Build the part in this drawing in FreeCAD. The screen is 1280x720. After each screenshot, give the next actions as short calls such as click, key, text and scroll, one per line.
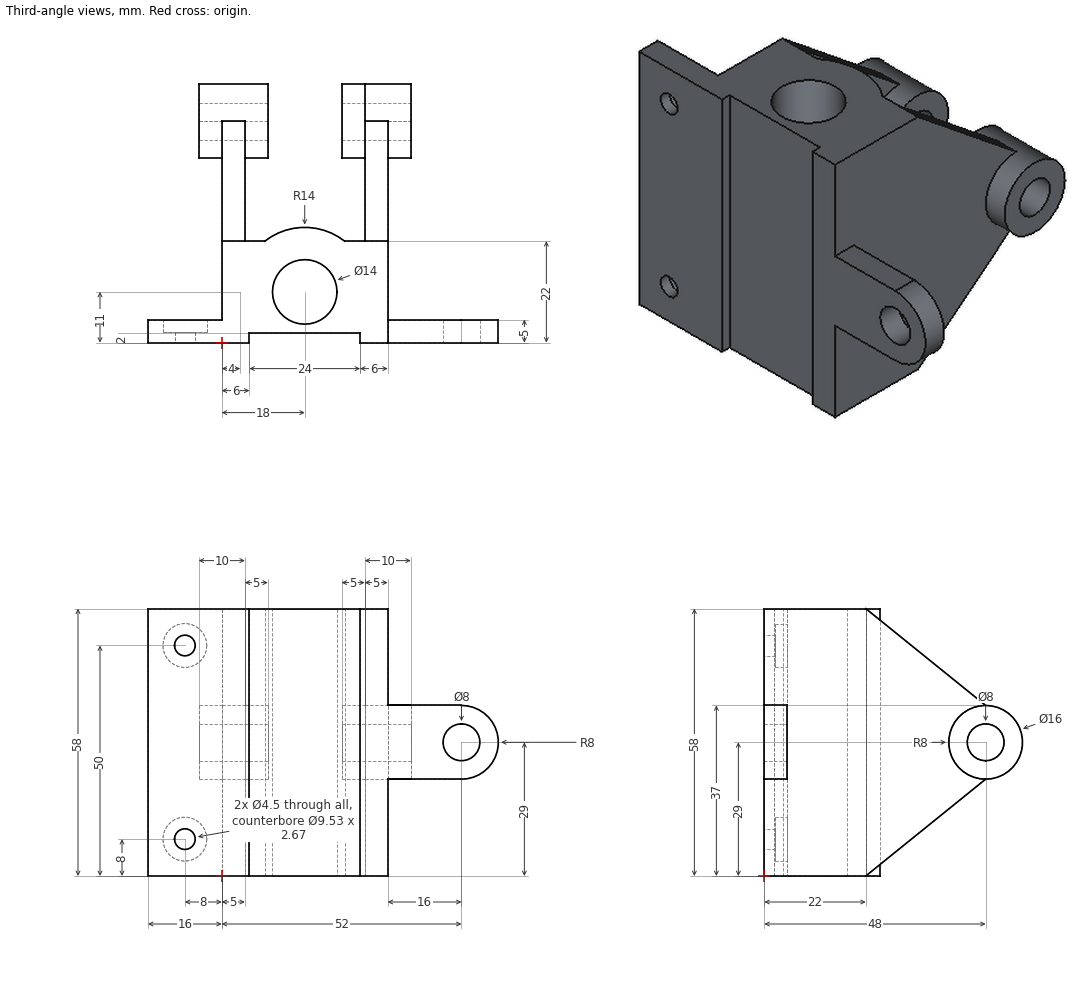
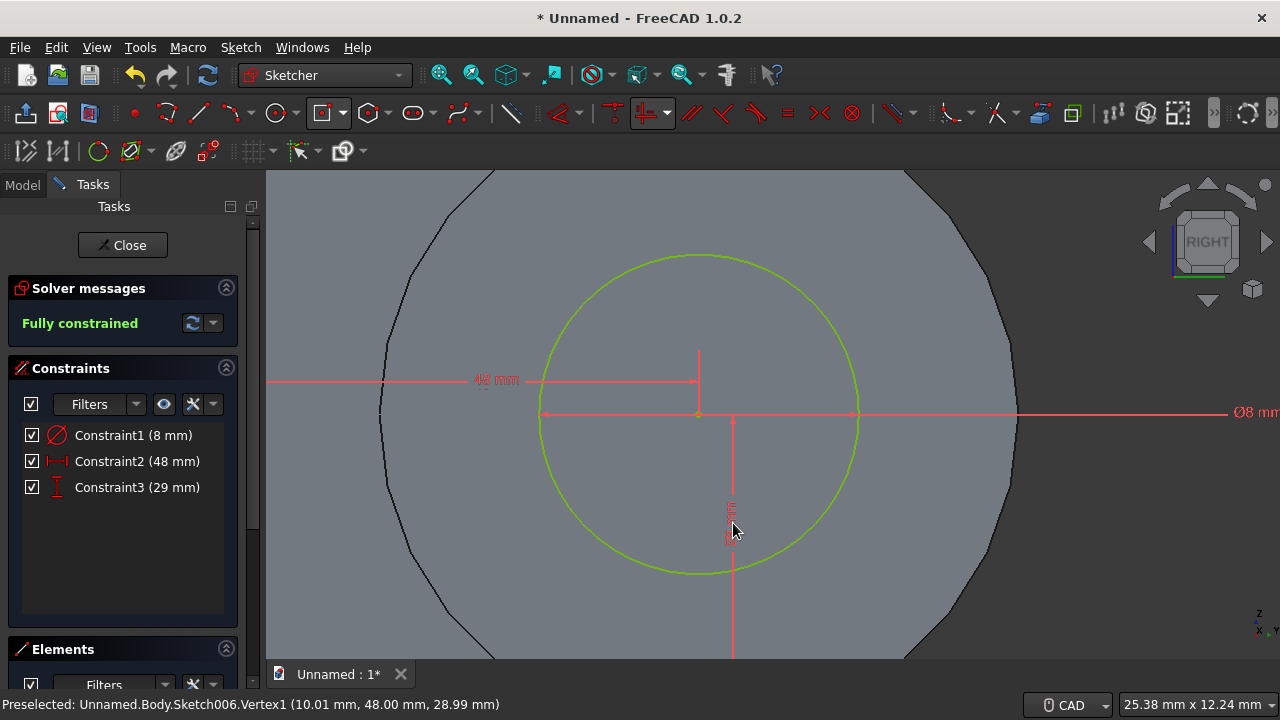
click(123, 245)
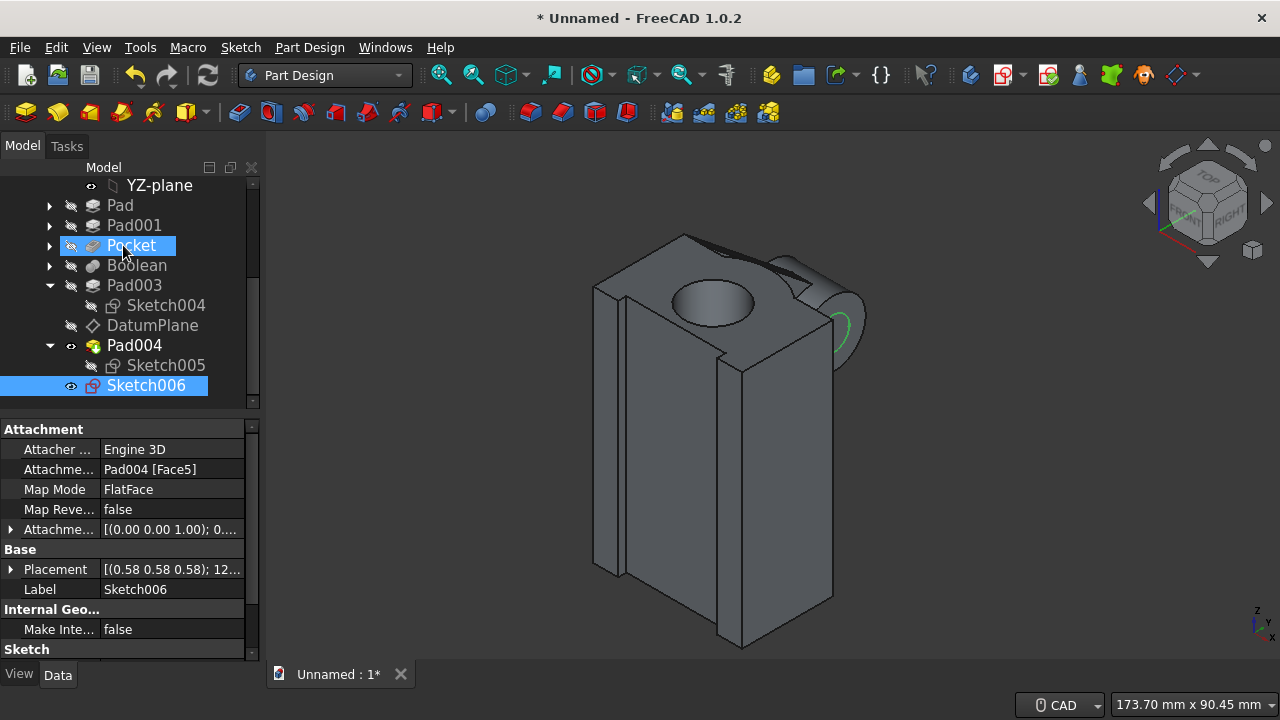
click(240, 112)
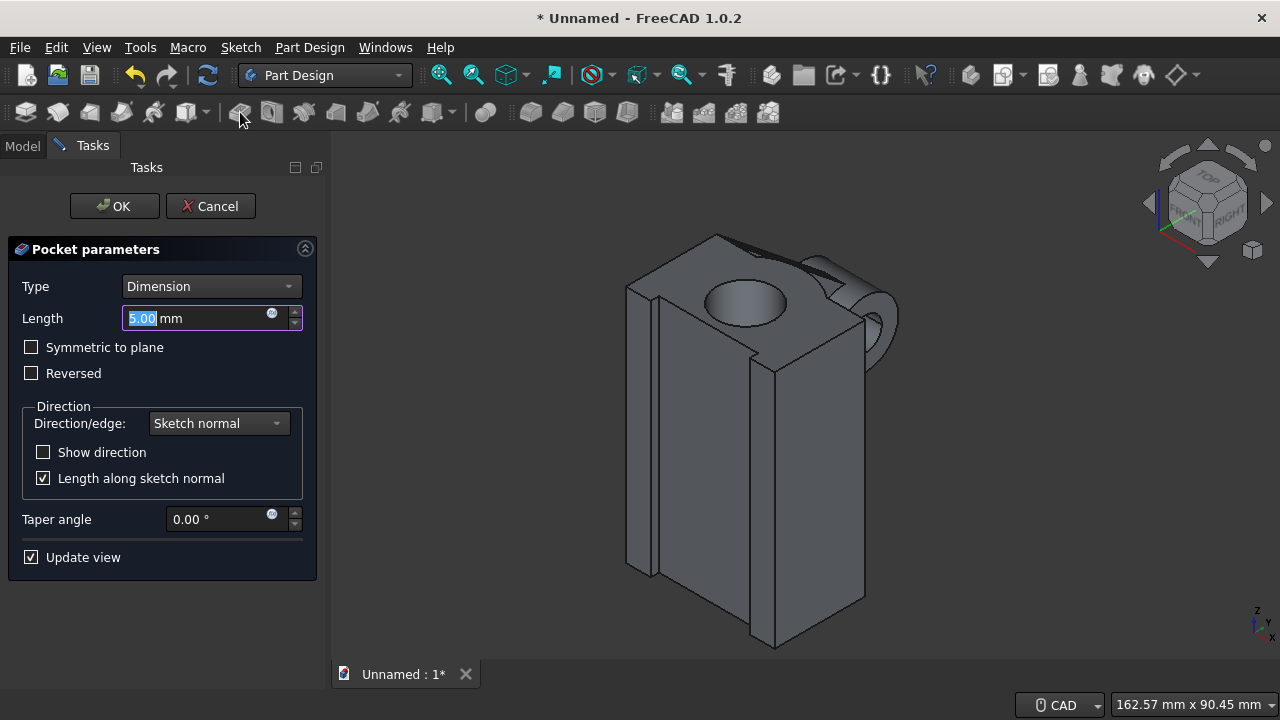
click(212, 286)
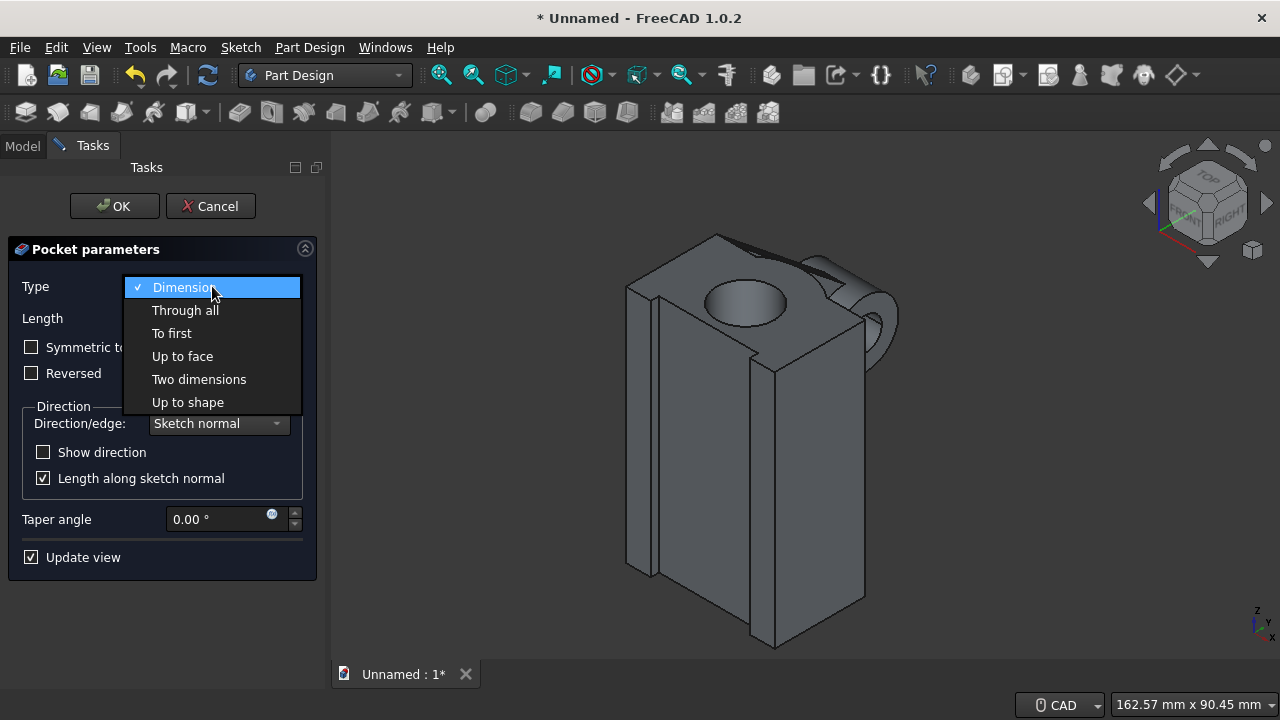
click(212, 310)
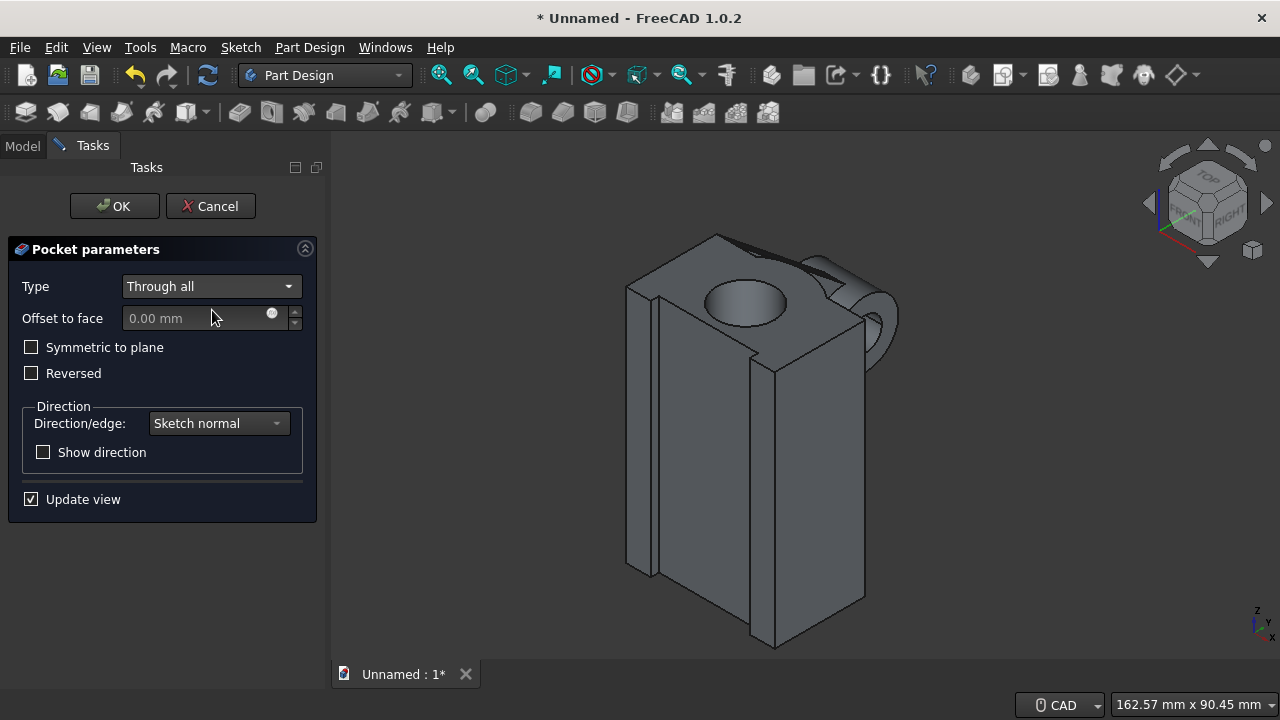
click(115, 206)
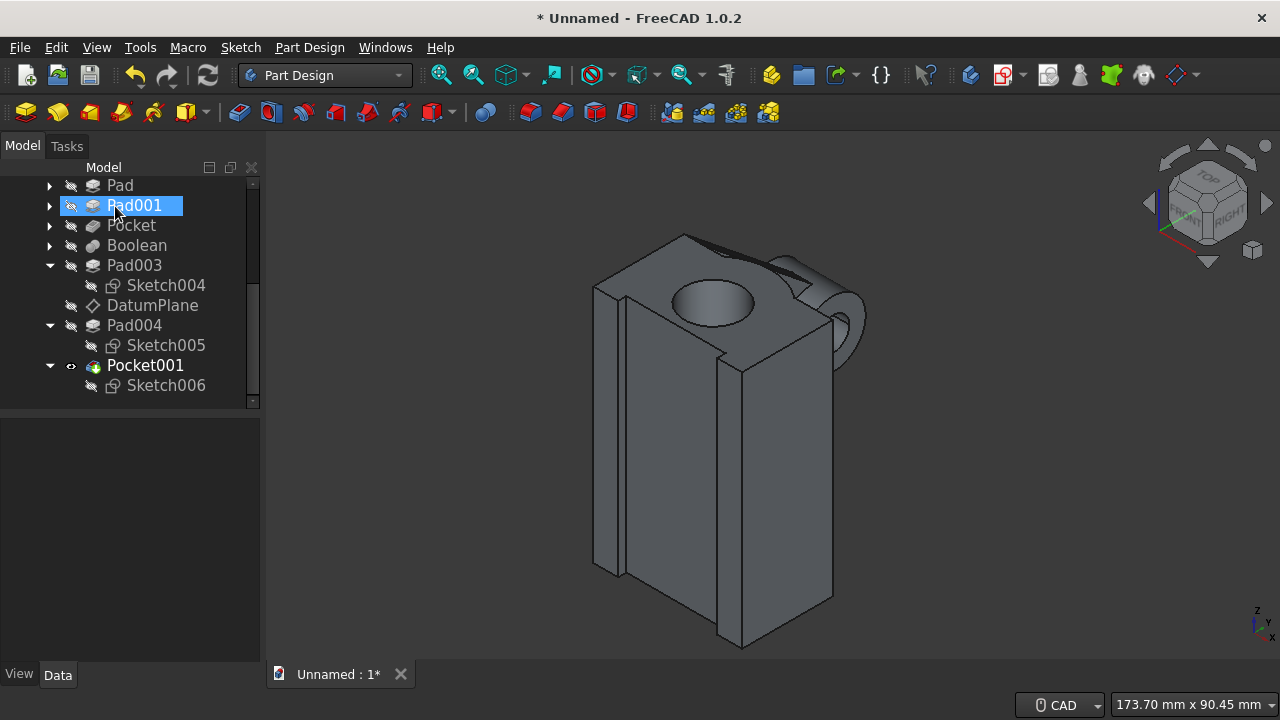
click(972, 76)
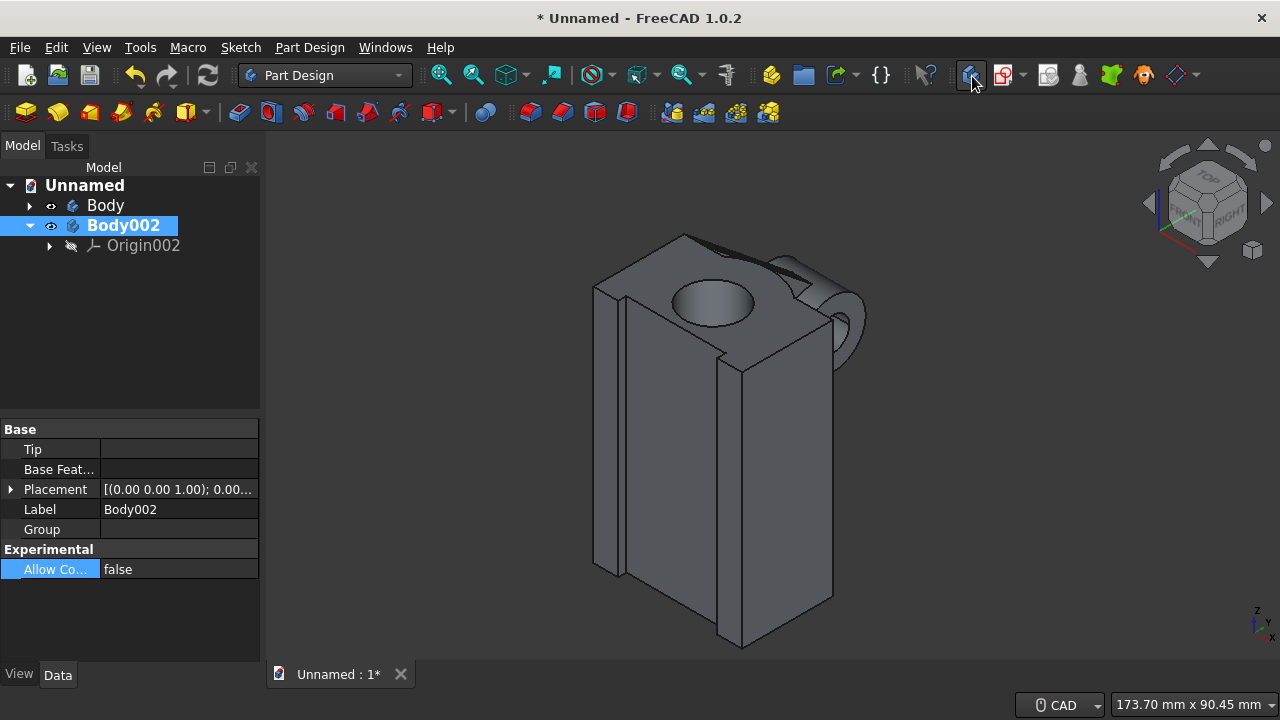
click(50, 246)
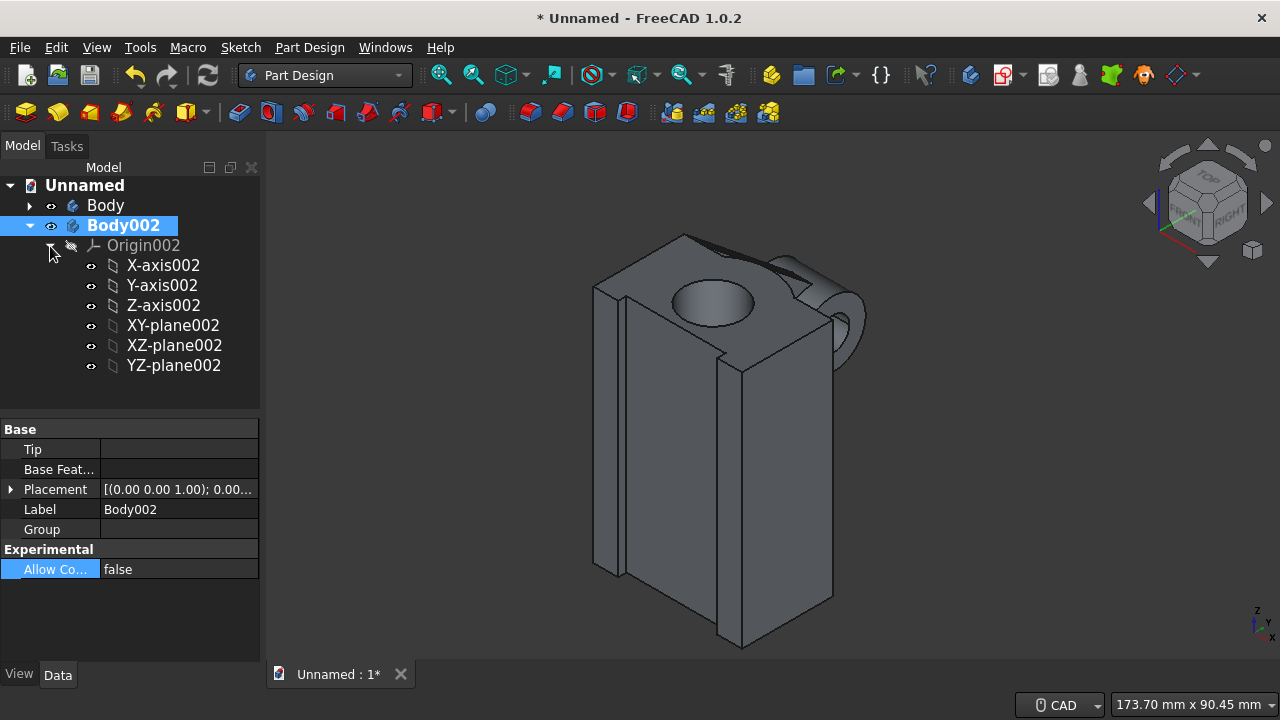
click(136, 366)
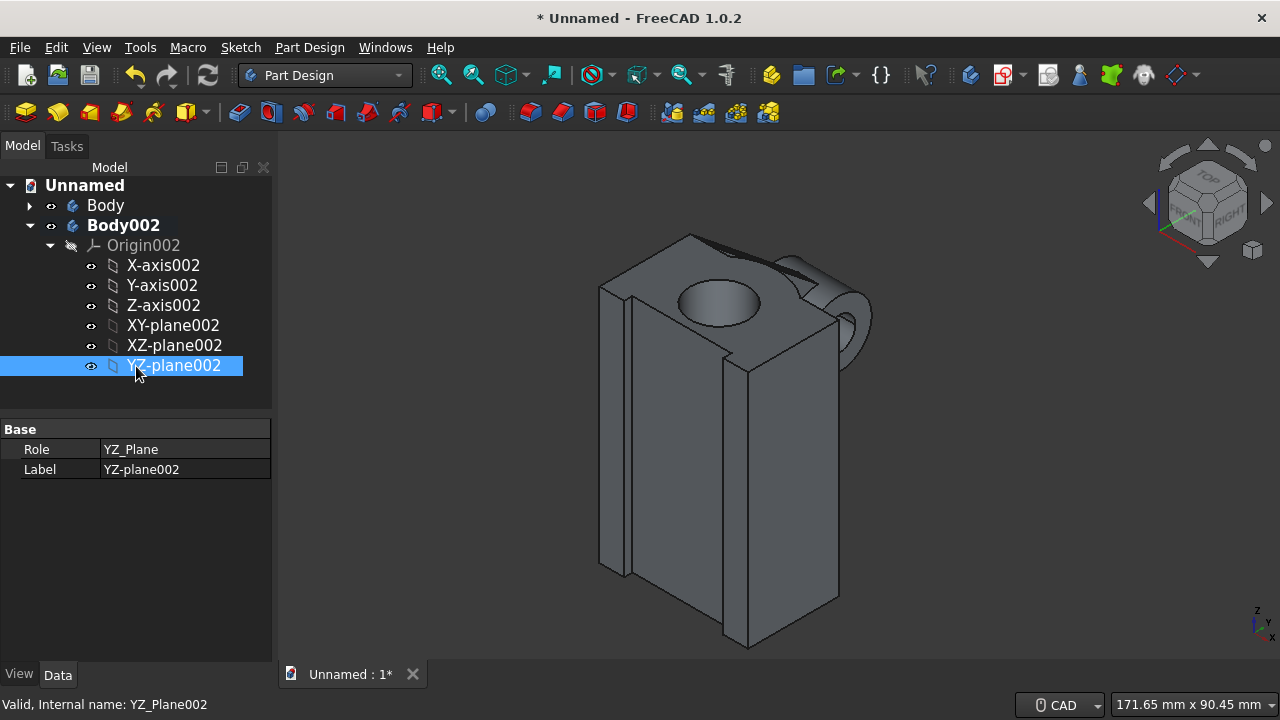
click(1176, 76)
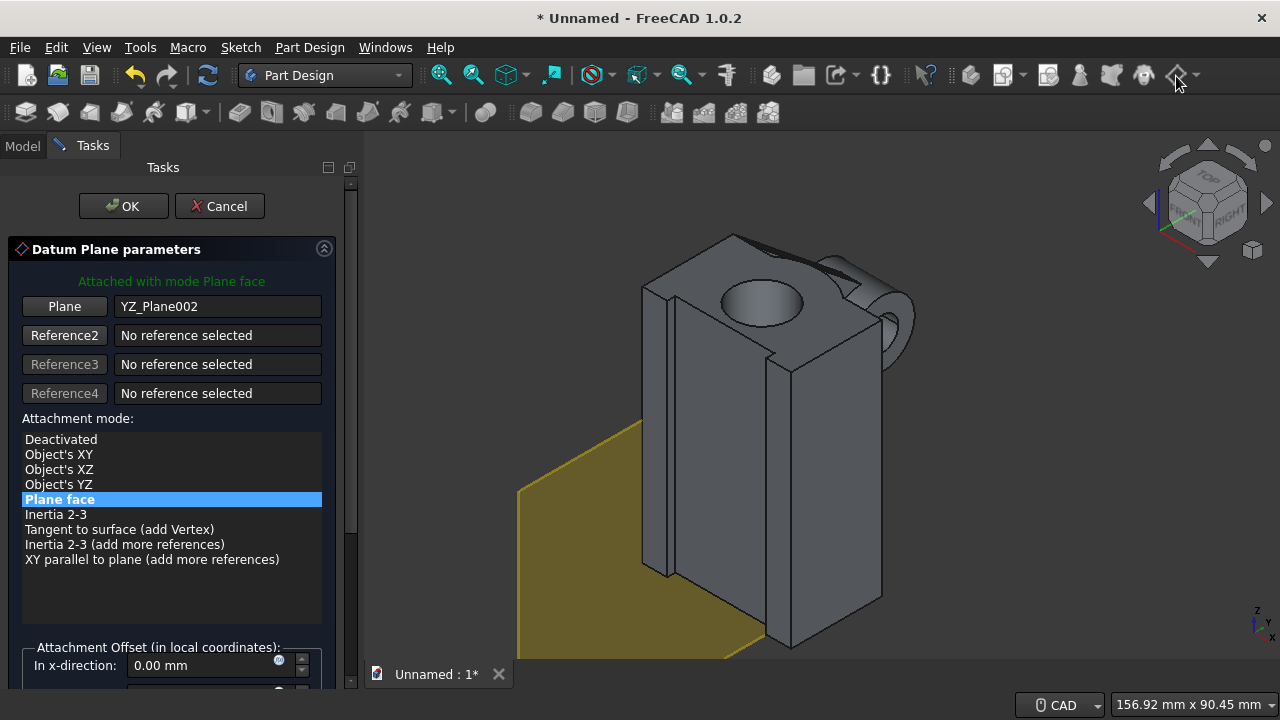
scroll(351, 432, down, 2)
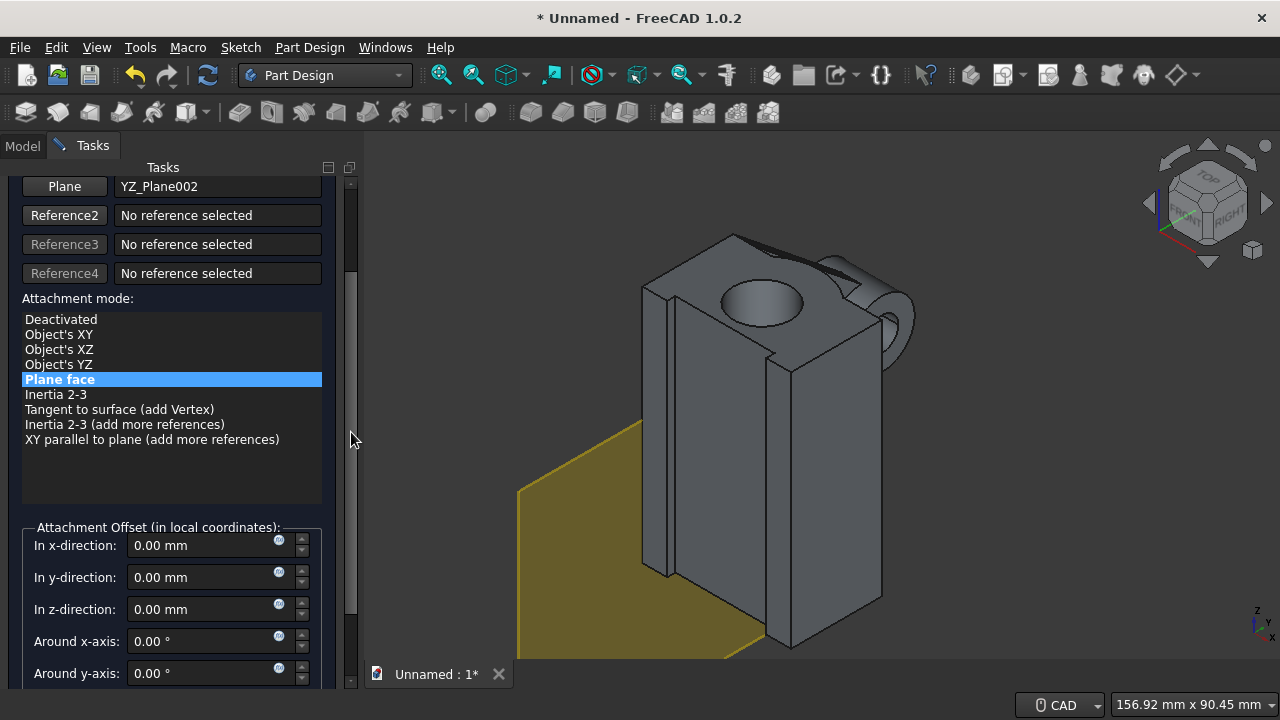
triple_click(210, 609)